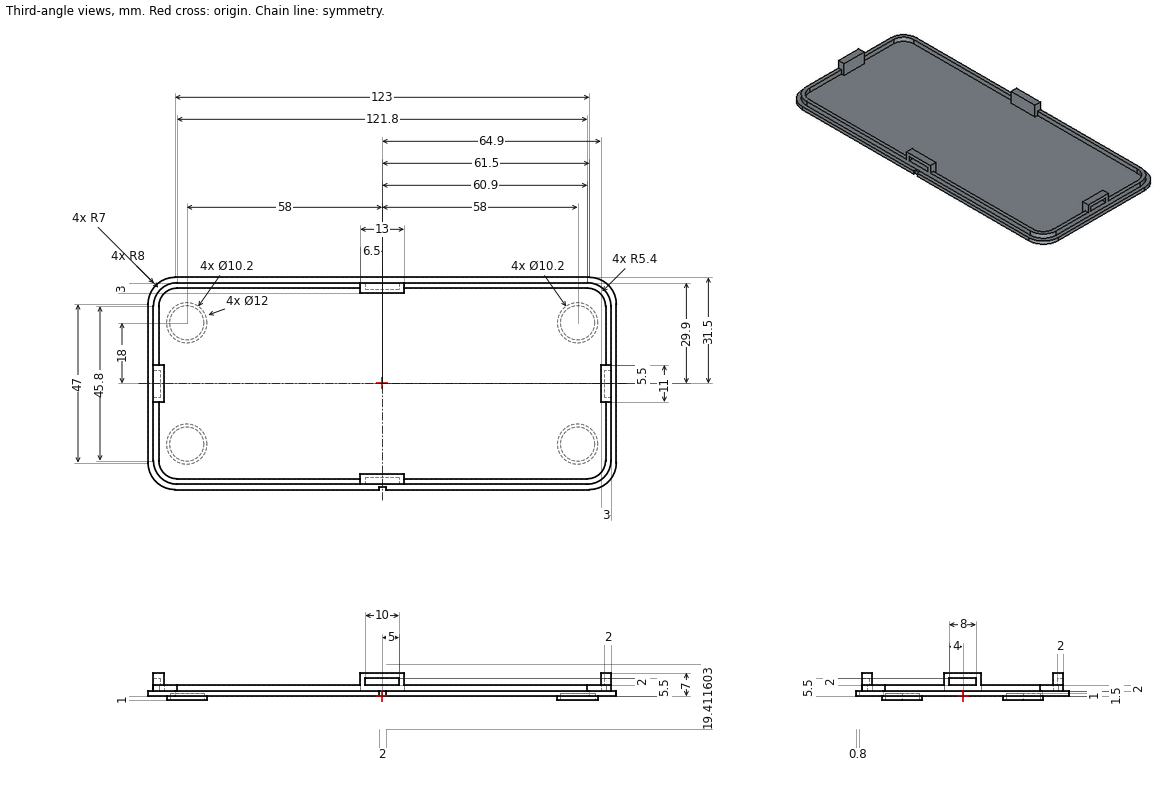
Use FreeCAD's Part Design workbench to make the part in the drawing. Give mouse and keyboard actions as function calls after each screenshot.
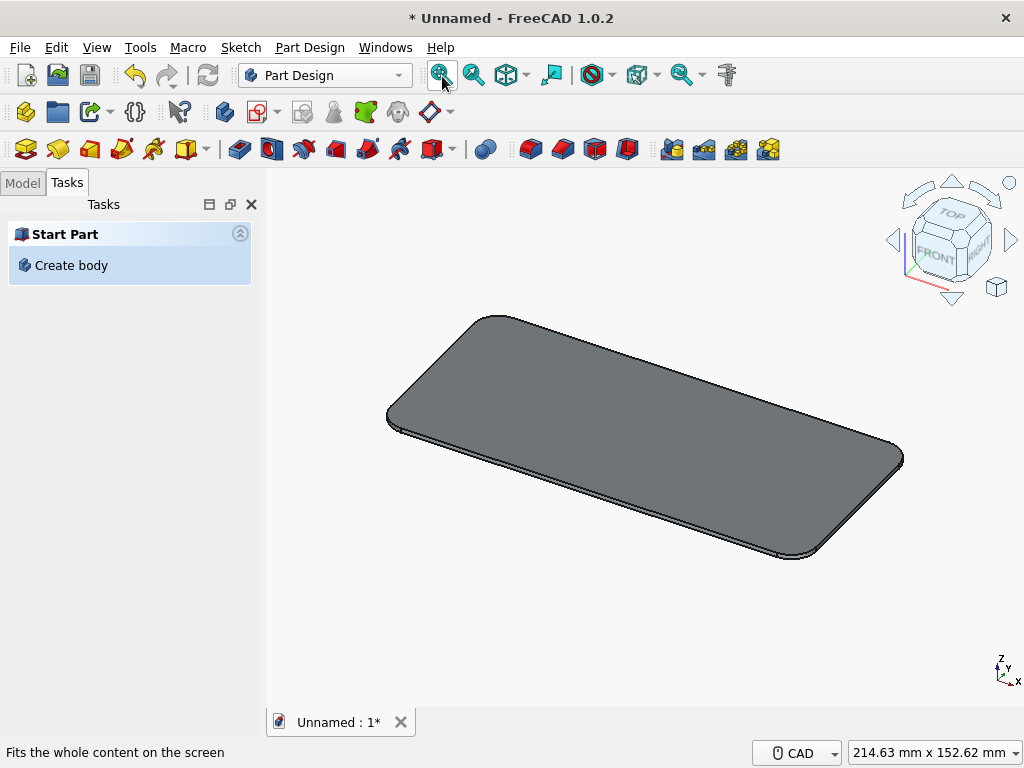
key(5)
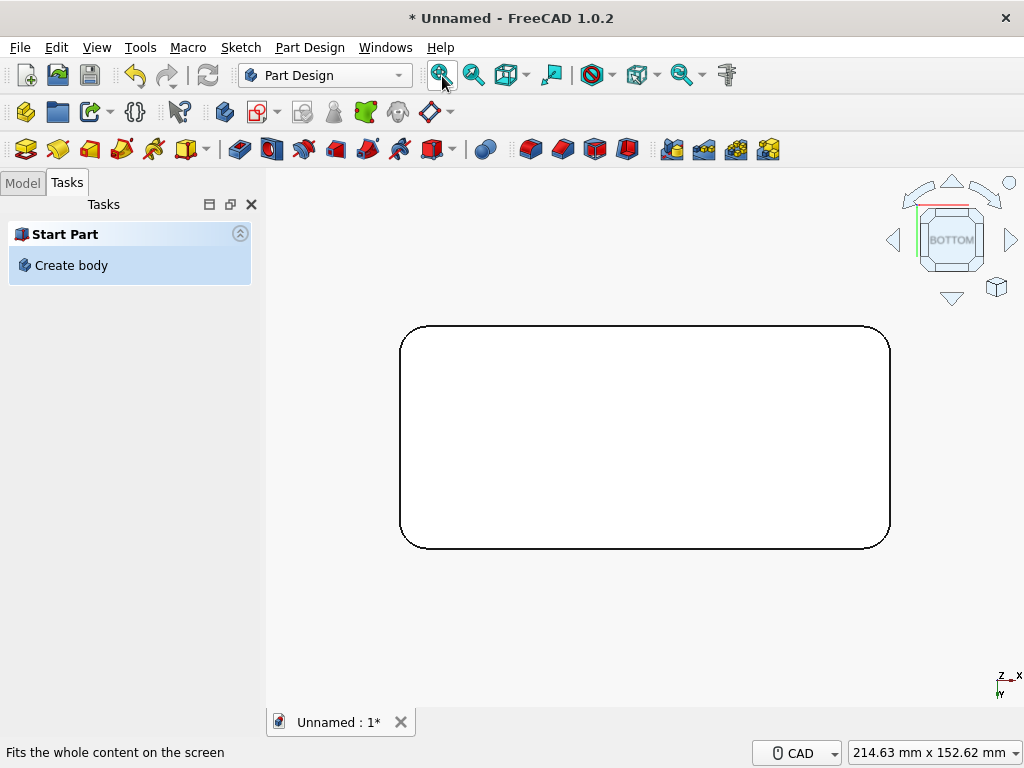
click(715, 436)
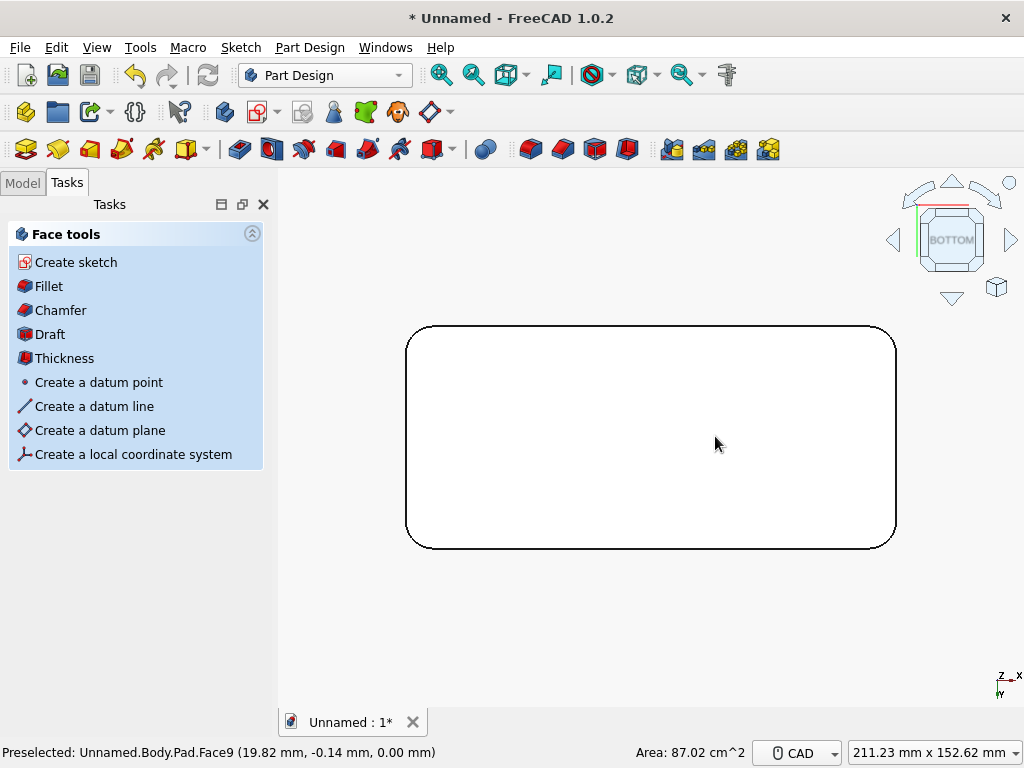
click(258, 112)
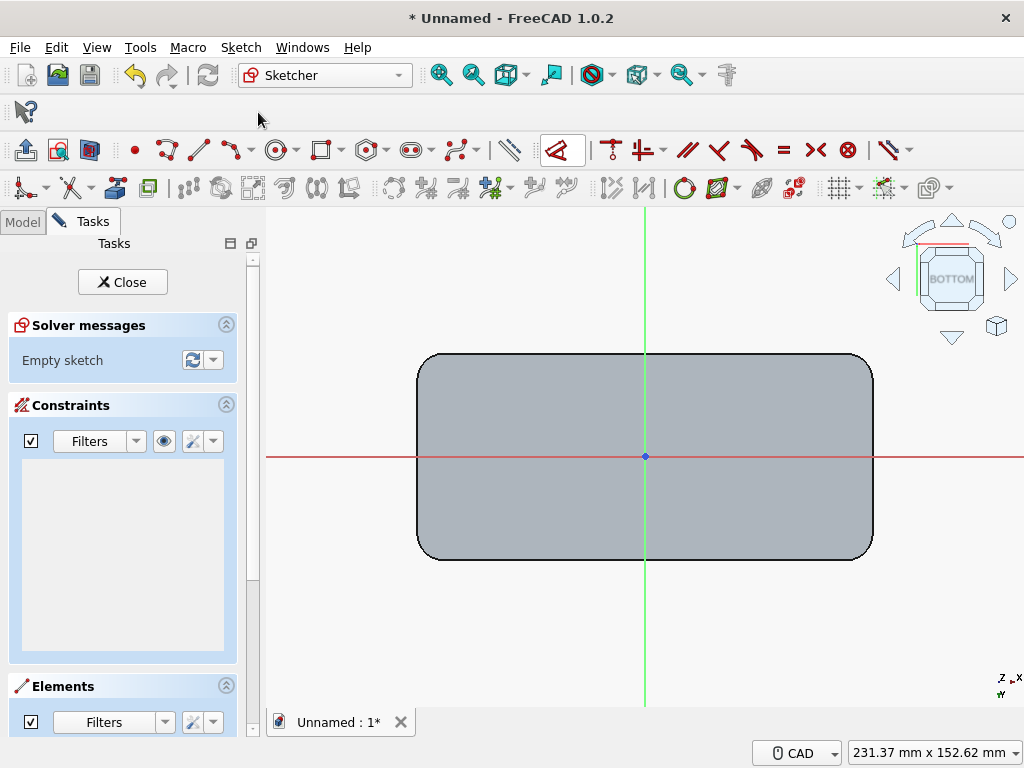
scroll(294, 457, down, 1)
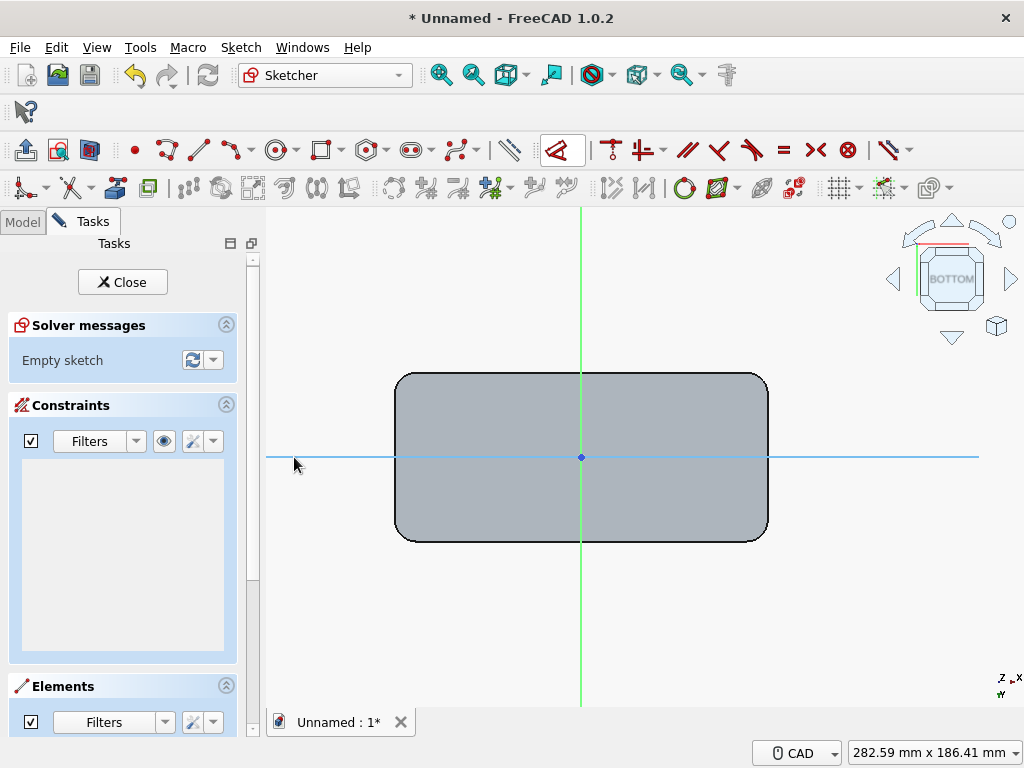
key(g)
key(c)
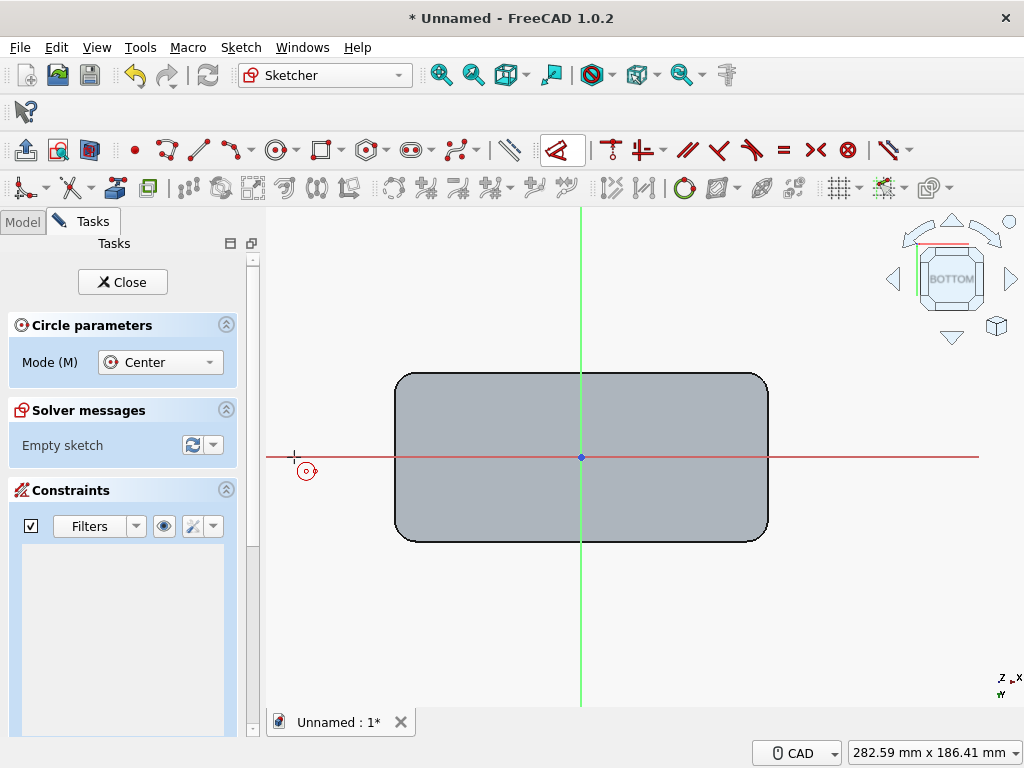
scroll(426, 505, up, 2)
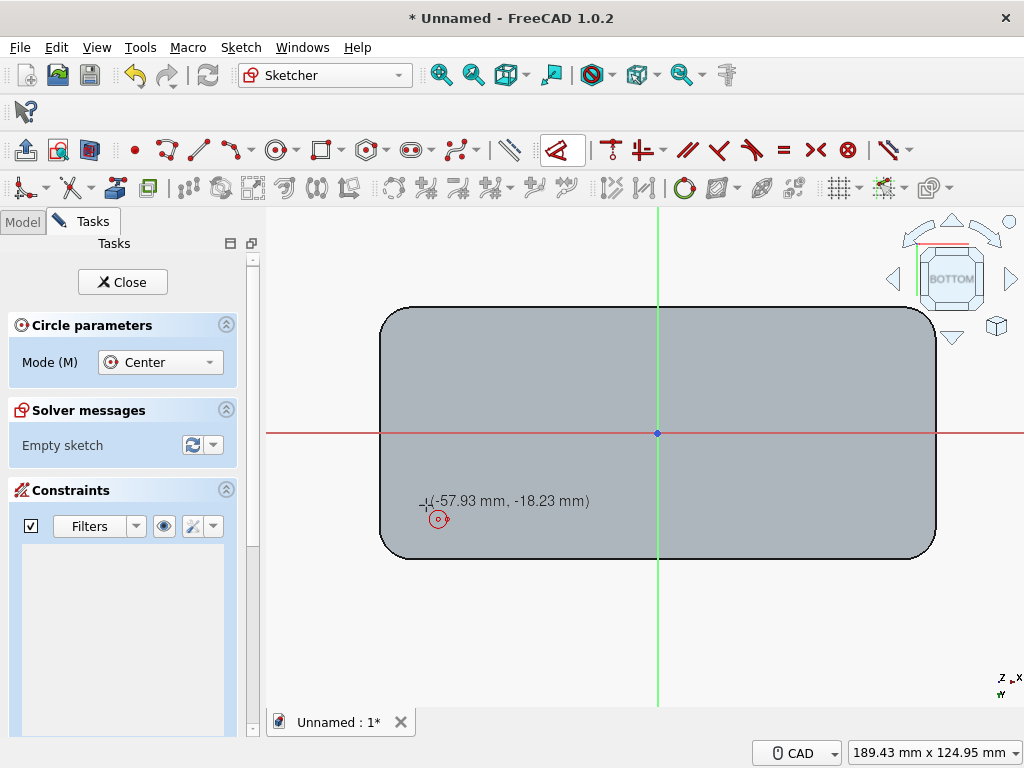
click(426, 505)
click(443, 488)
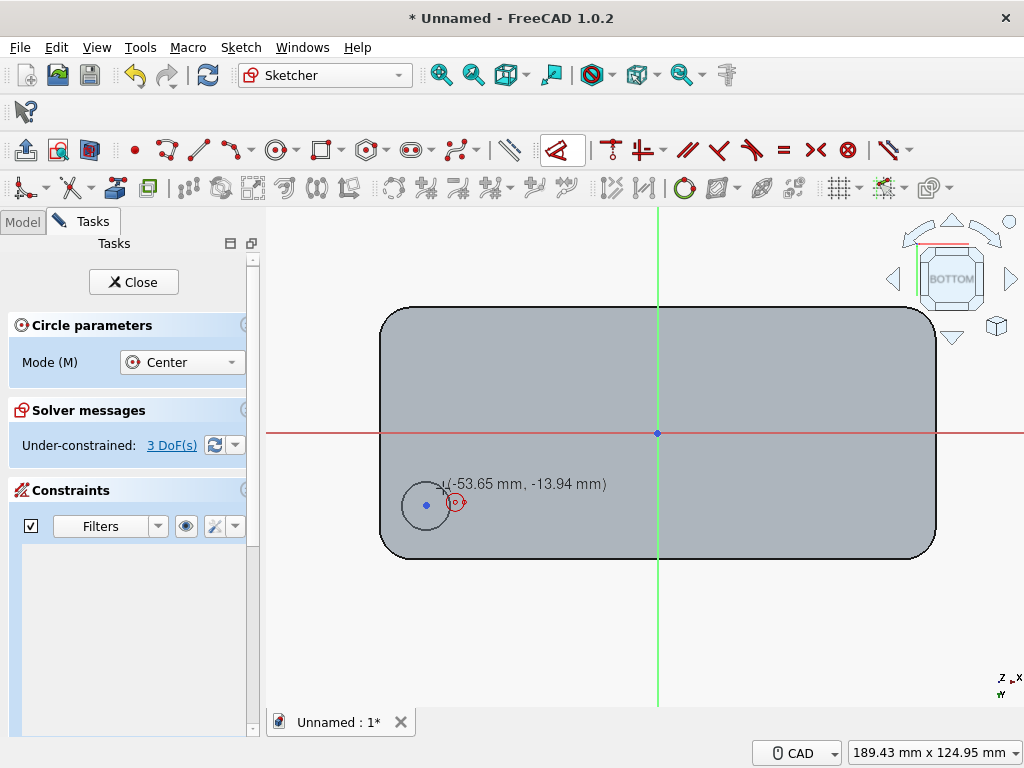
scroll(294, 564, down, 1)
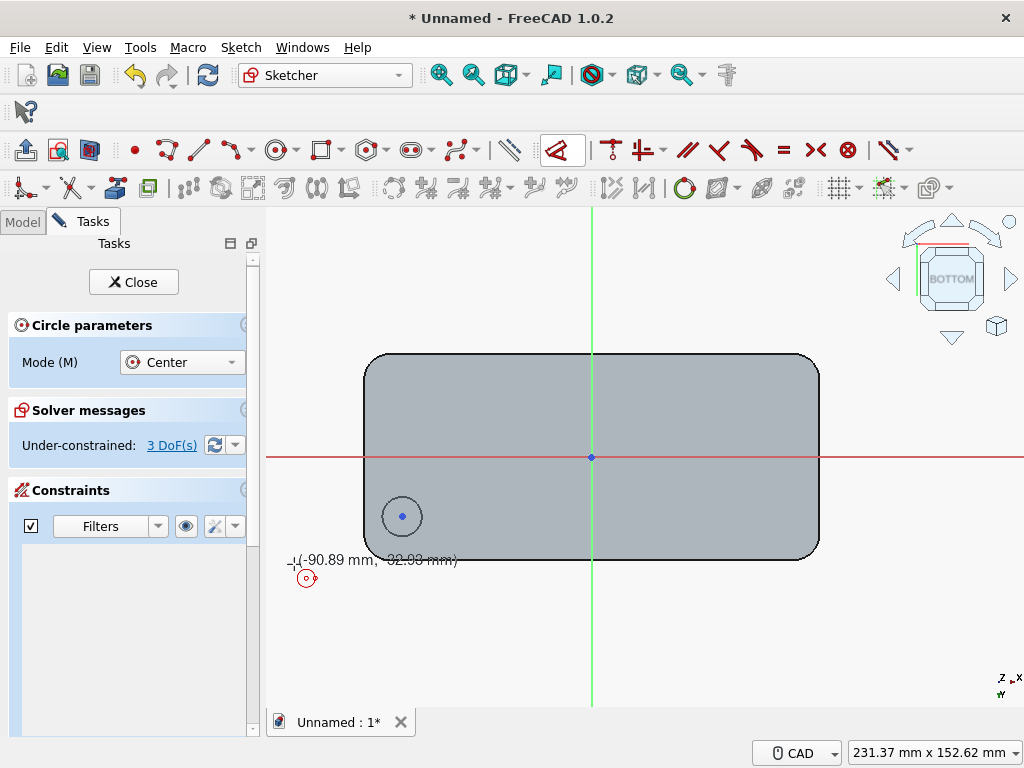
click(782, 516)
click(796, 502)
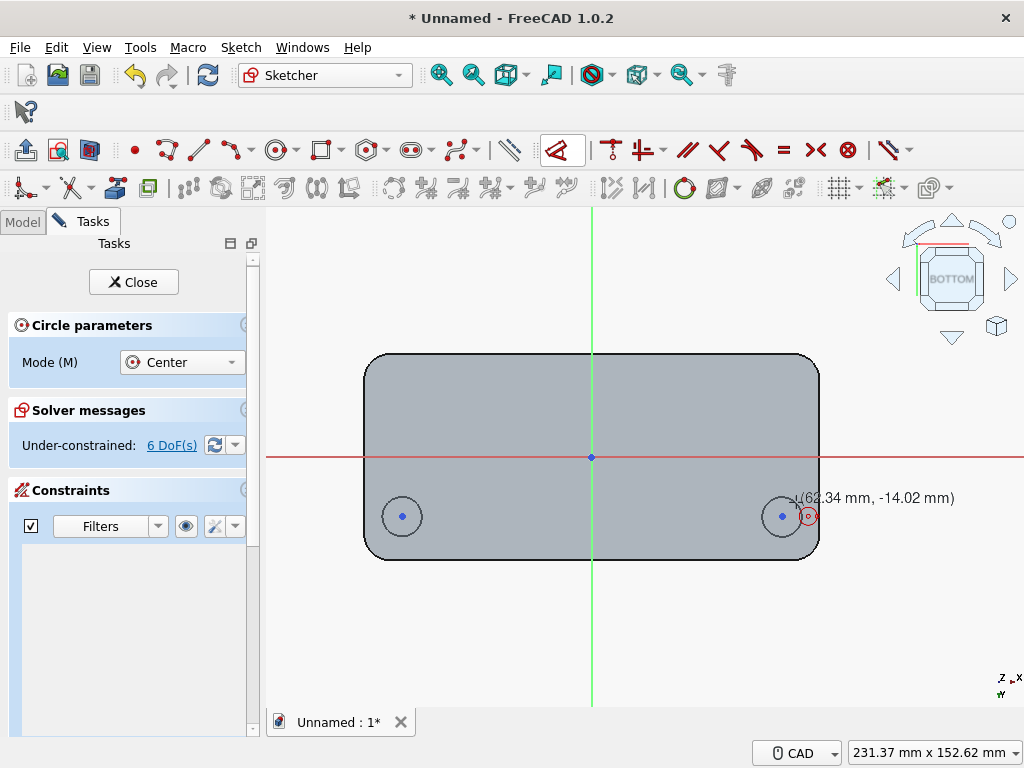
click(402, 398)
click(416, 384)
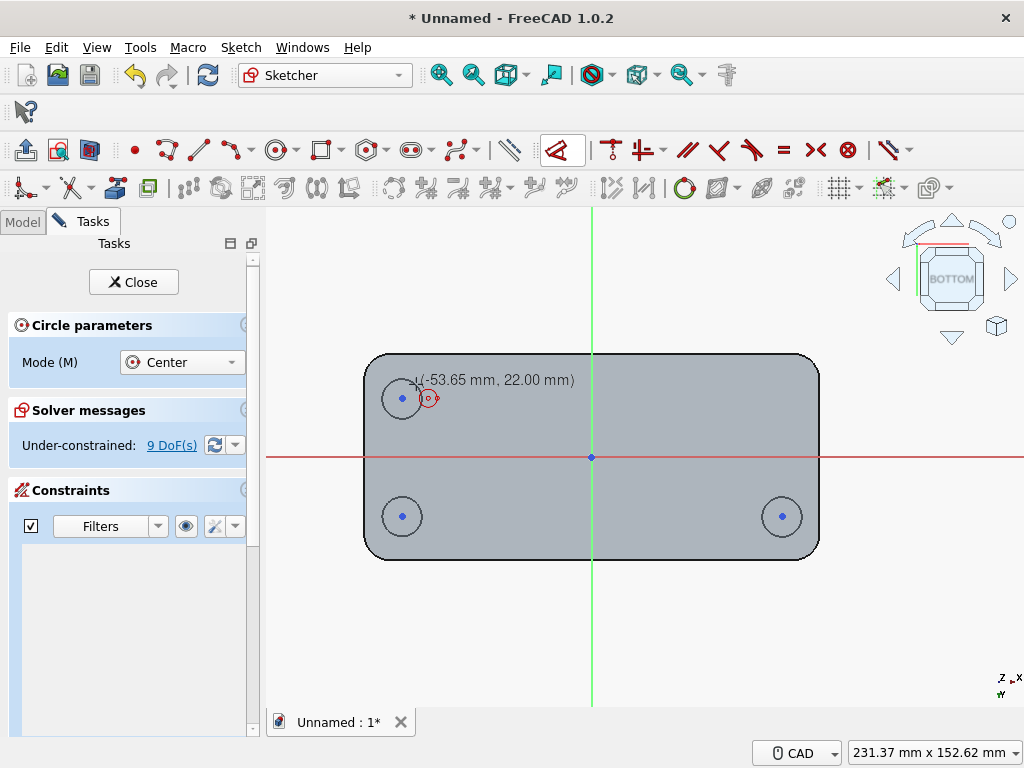
click(782, 398)
click(796, 384)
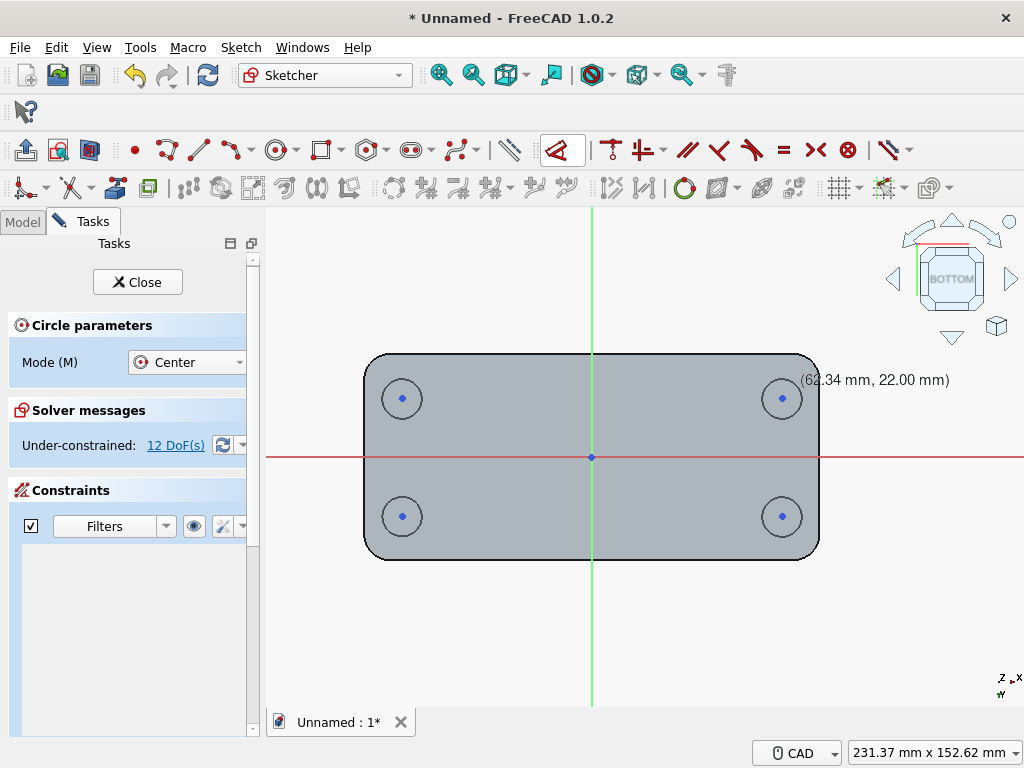
scroll(402, 516, up, 2)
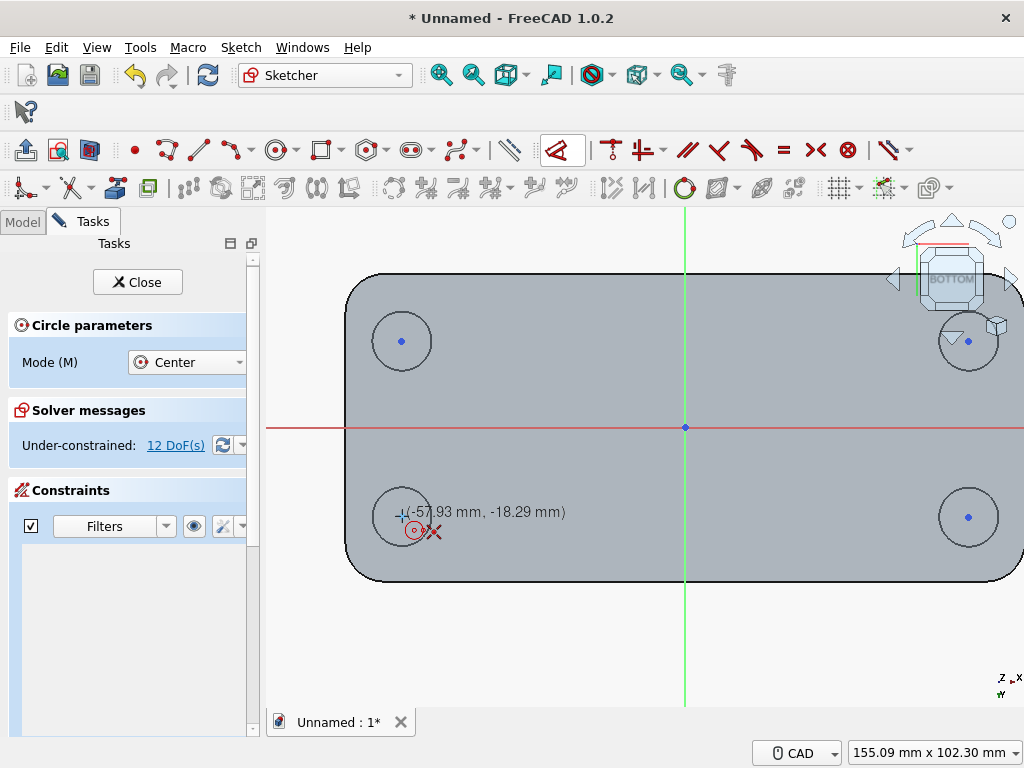
click(402, 517)